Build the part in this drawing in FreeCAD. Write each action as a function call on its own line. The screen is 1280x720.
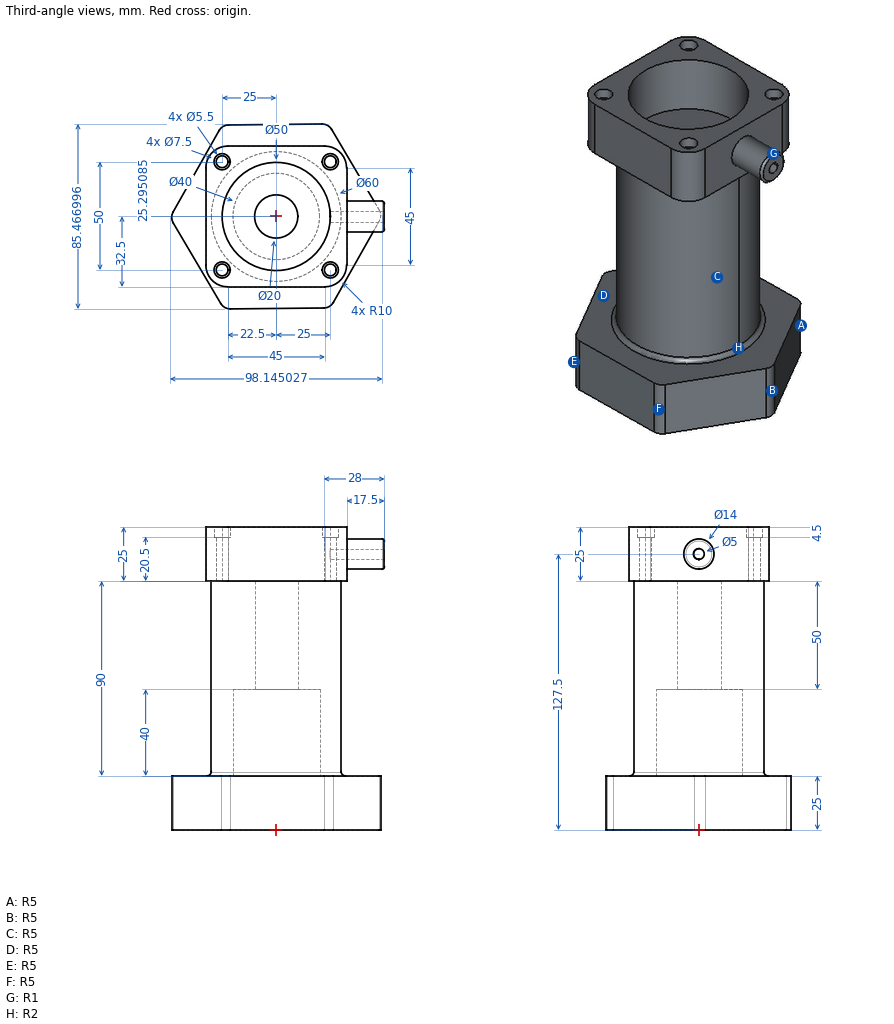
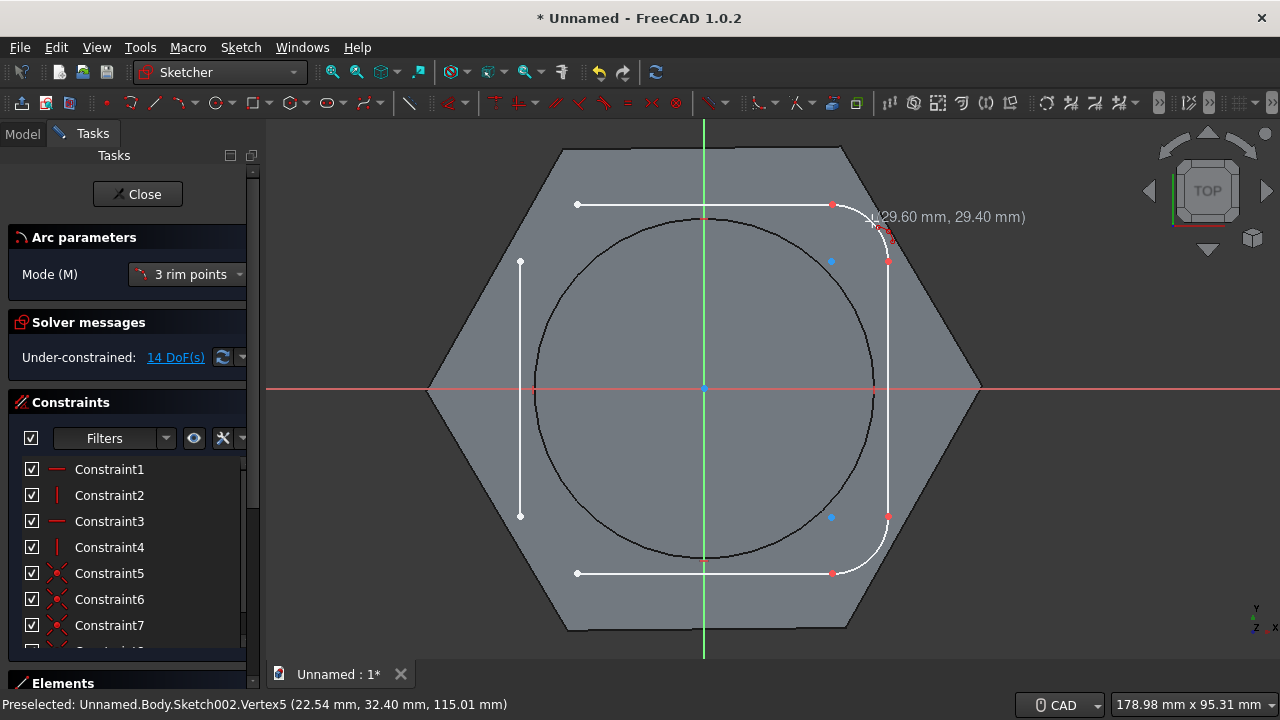
click(577, 205)
click(520, 262)
click(537, 221)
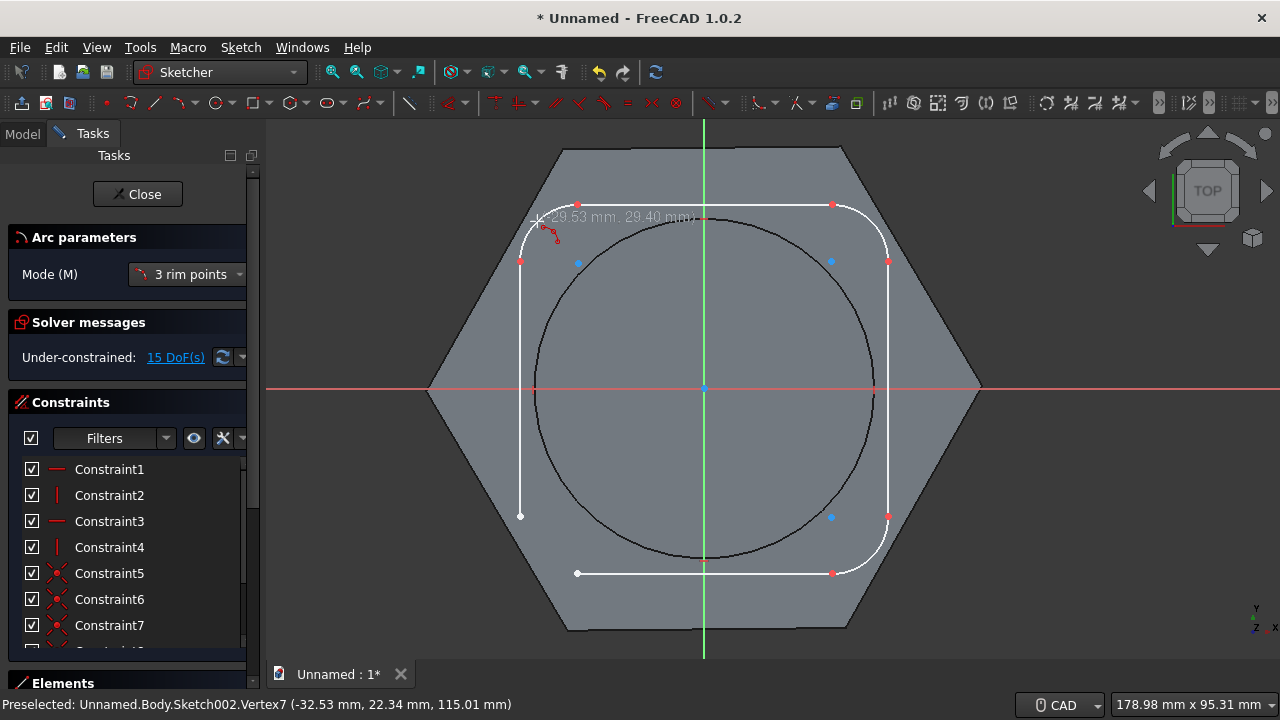
click(520, 517)
click(577, 574)
click(537, 556)
key(Escape)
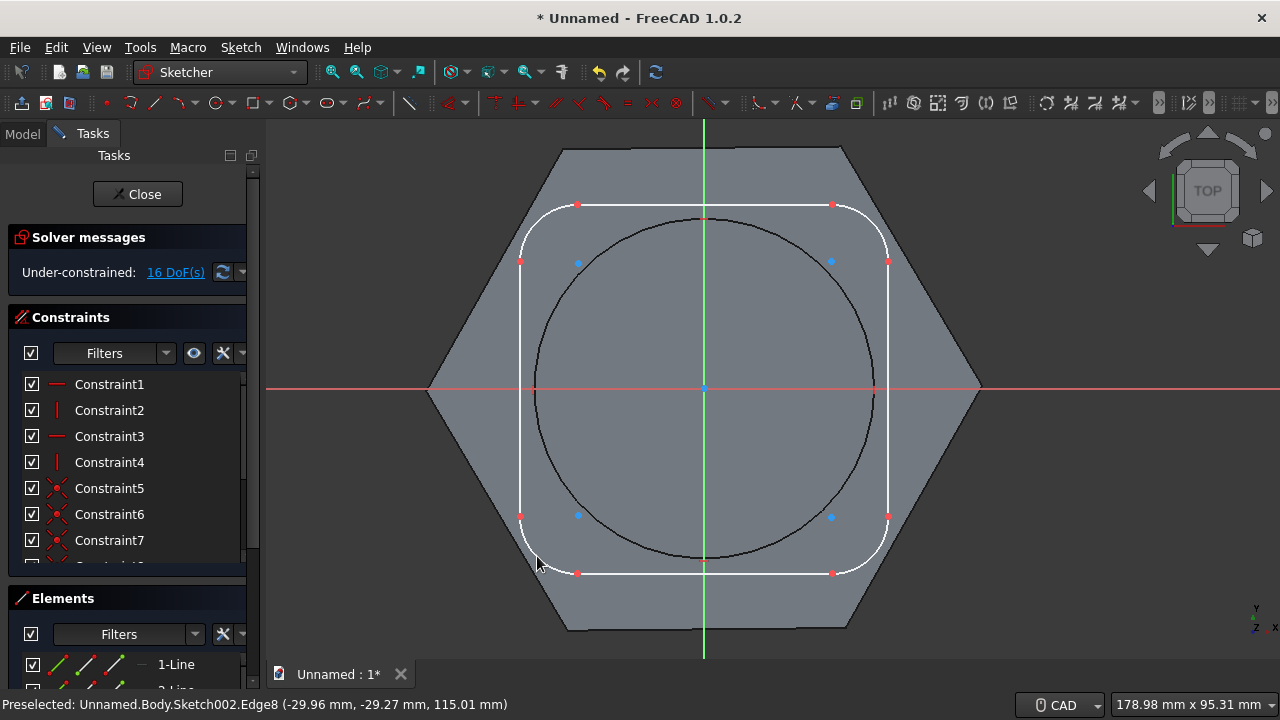
click(653, 574)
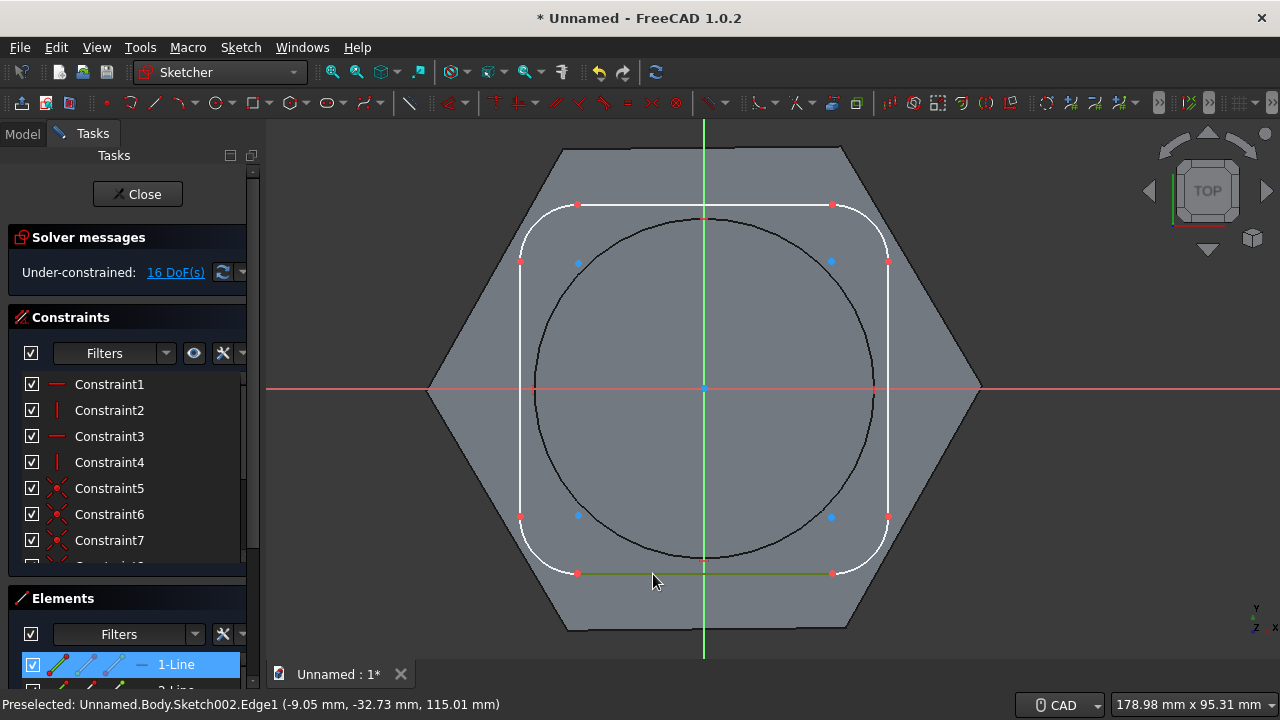
click(858, 568)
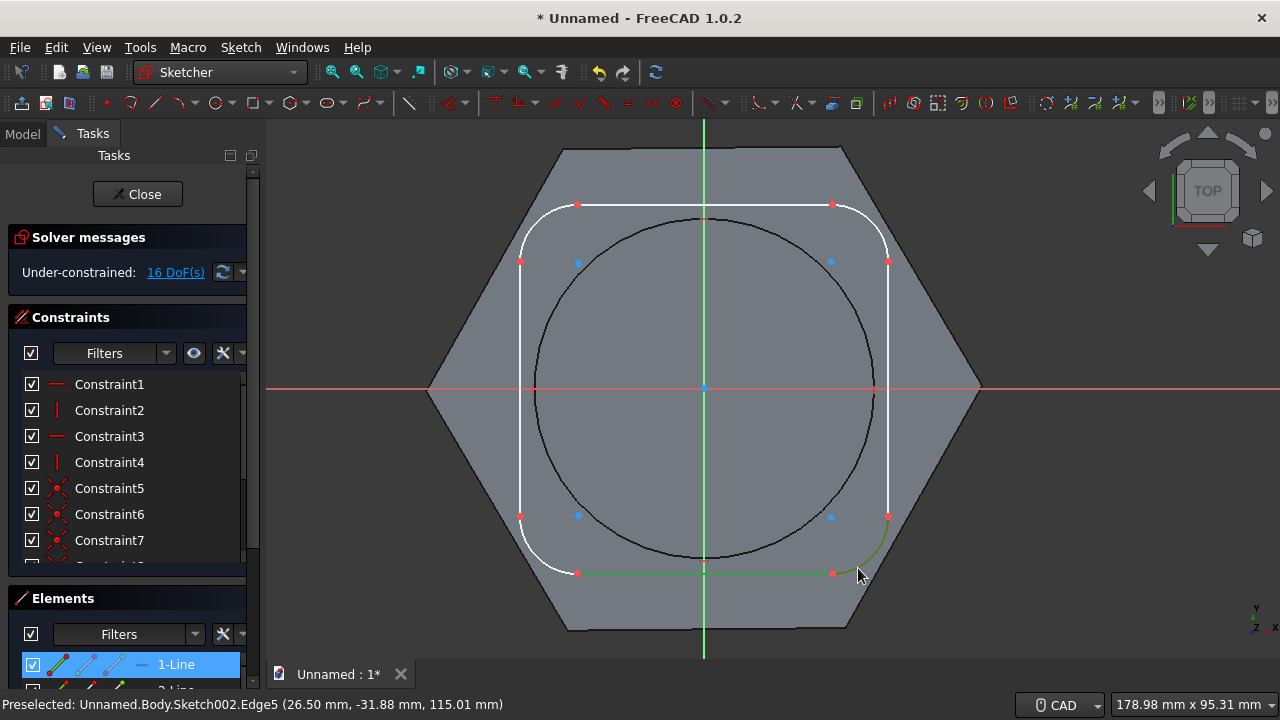
click(604, 104)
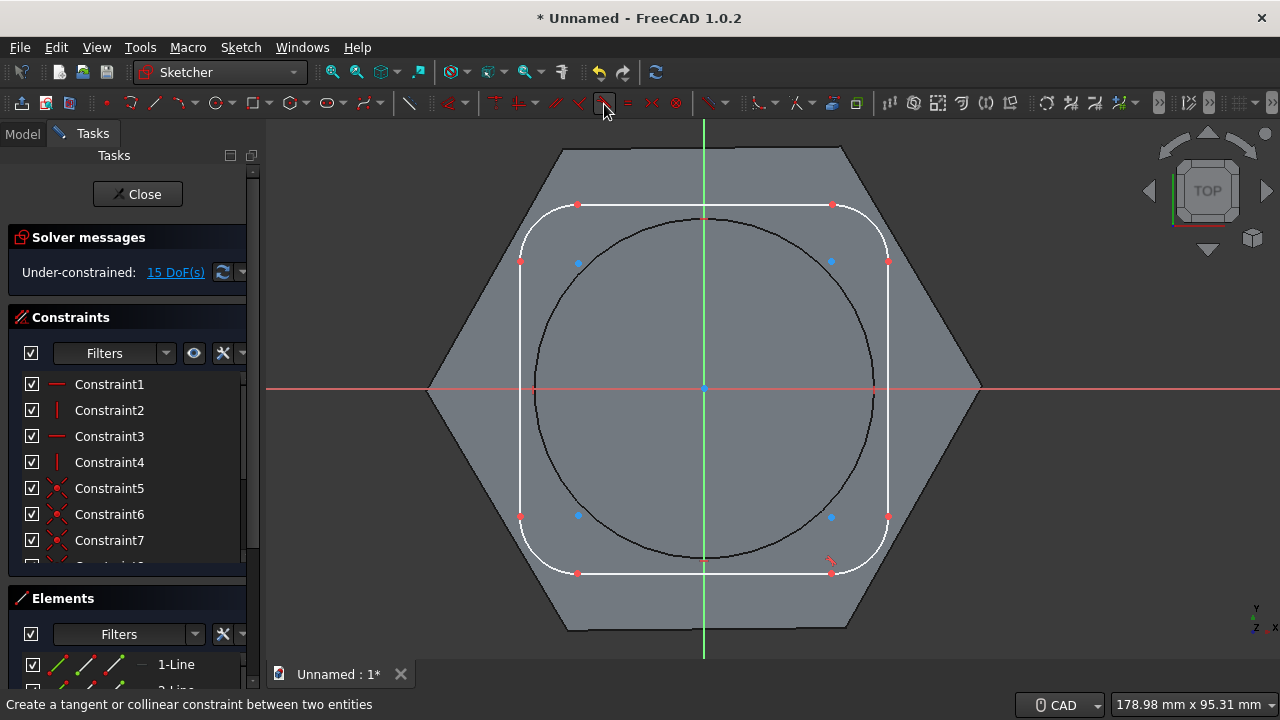
click(653, 574)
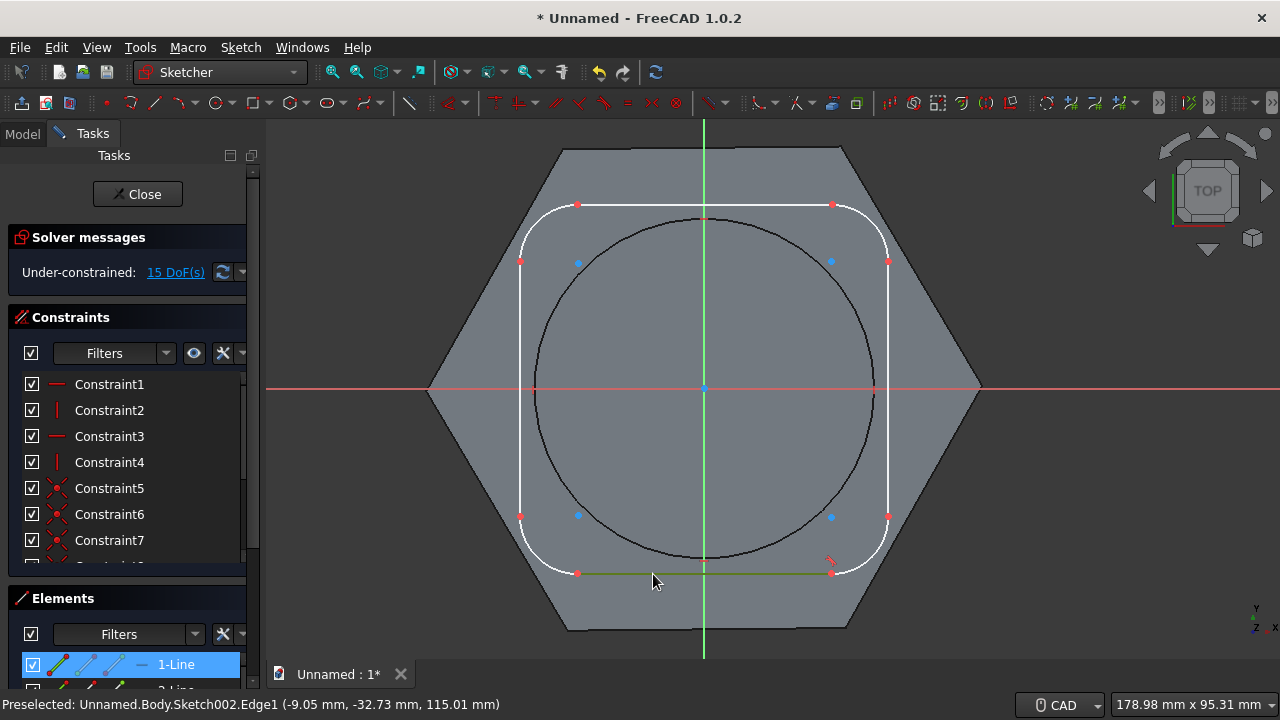
click(527, 543)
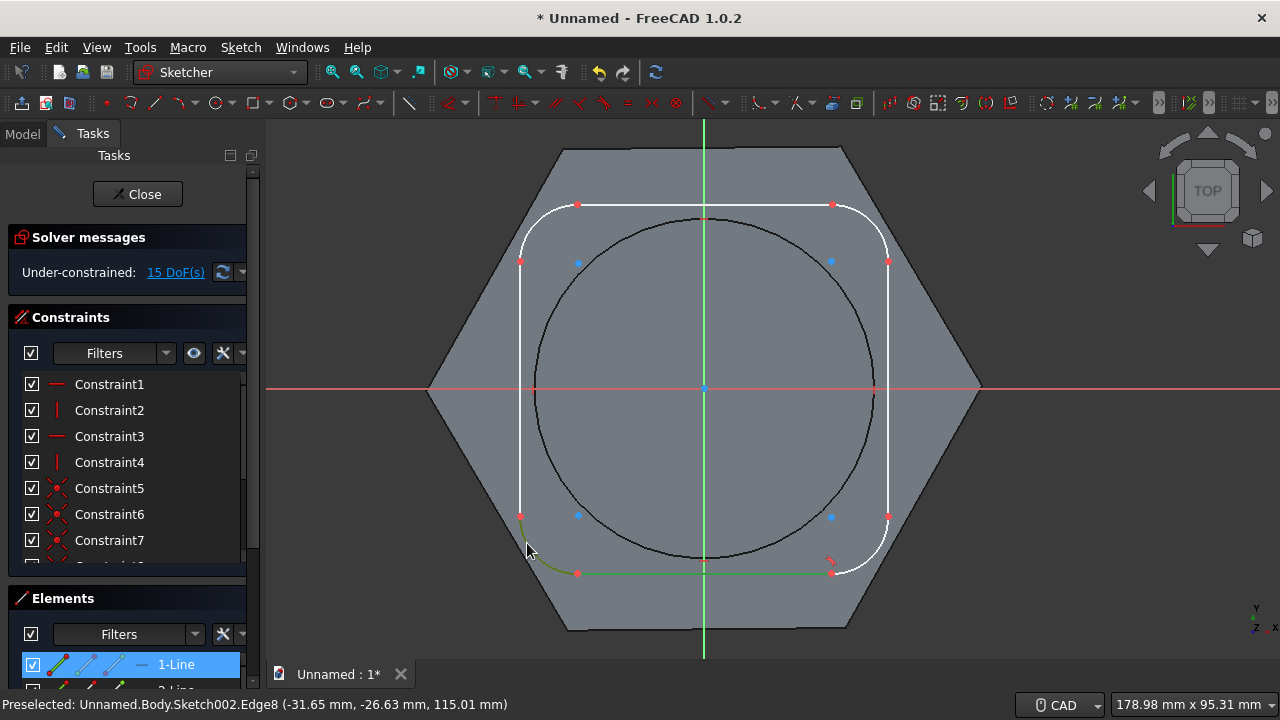
click(604, 104)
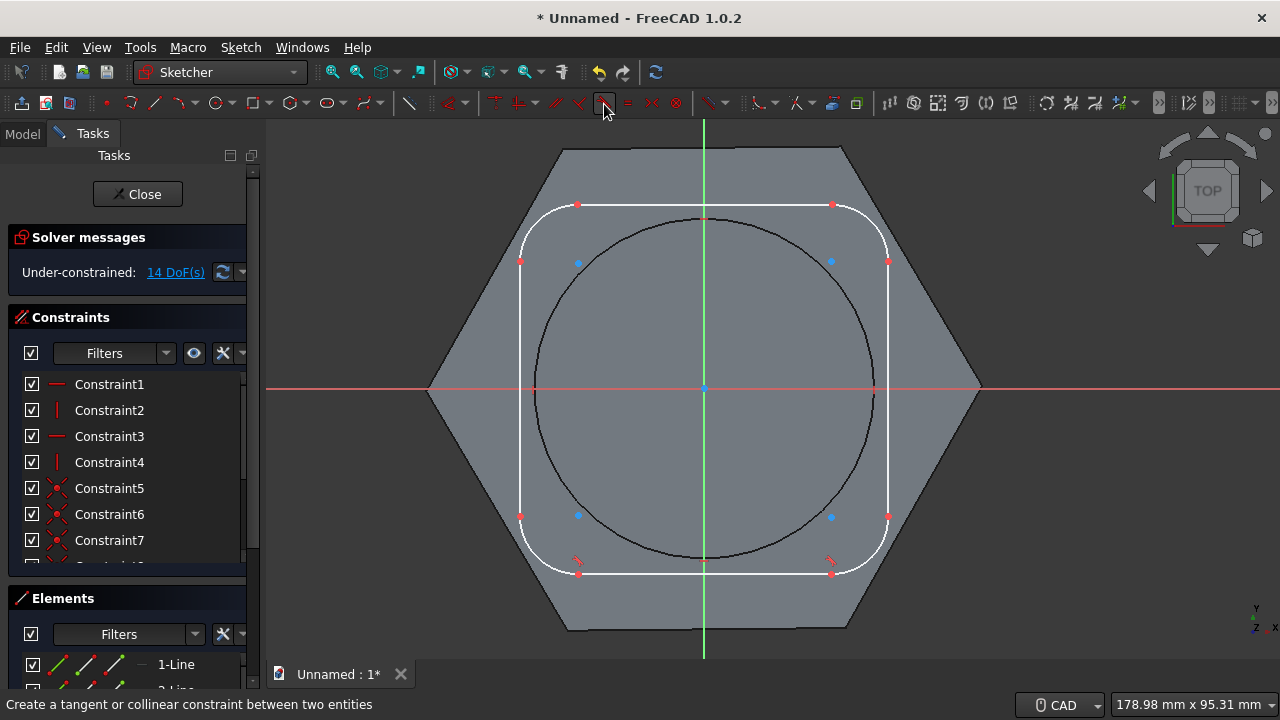
click(888, 441)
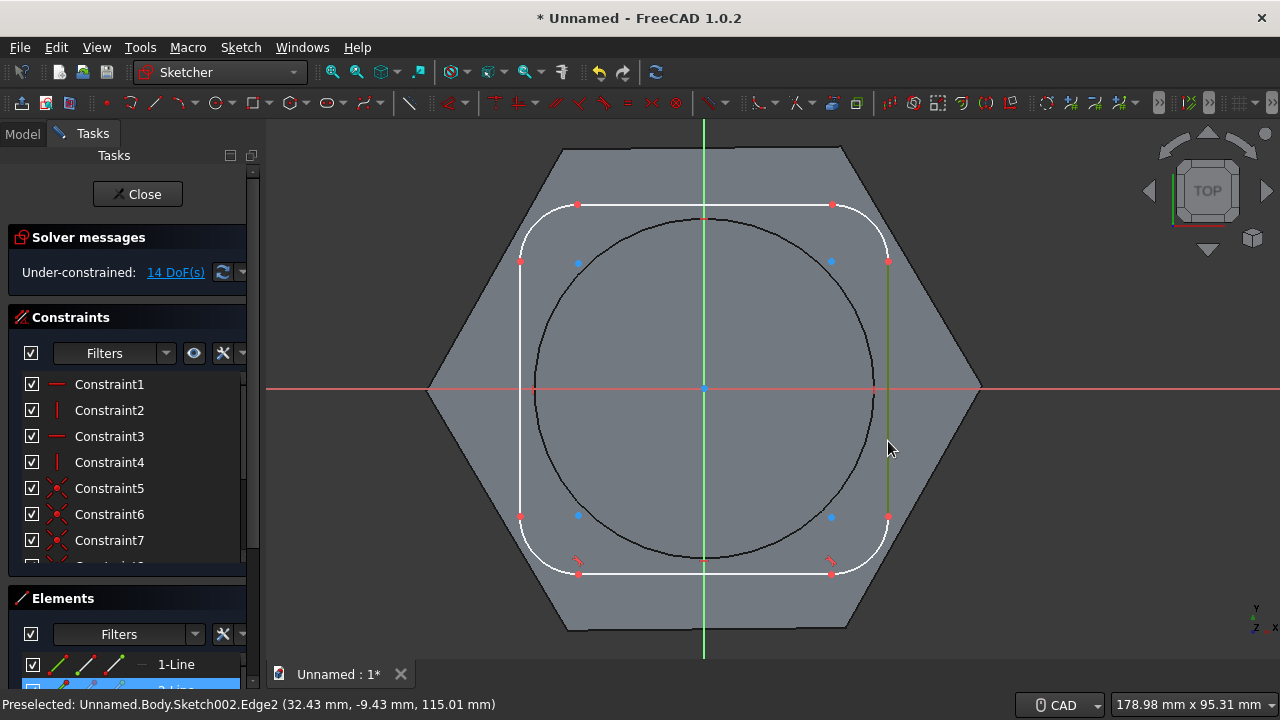
click(857, 568)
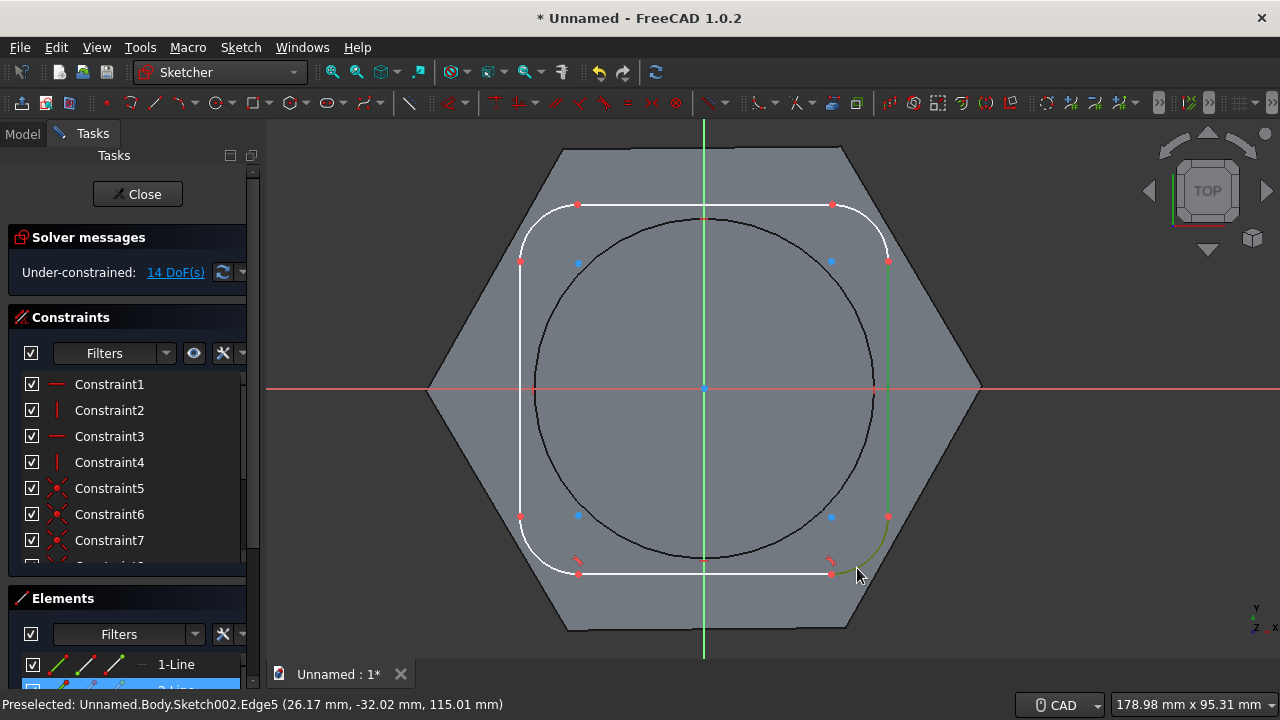
click(604, 104)